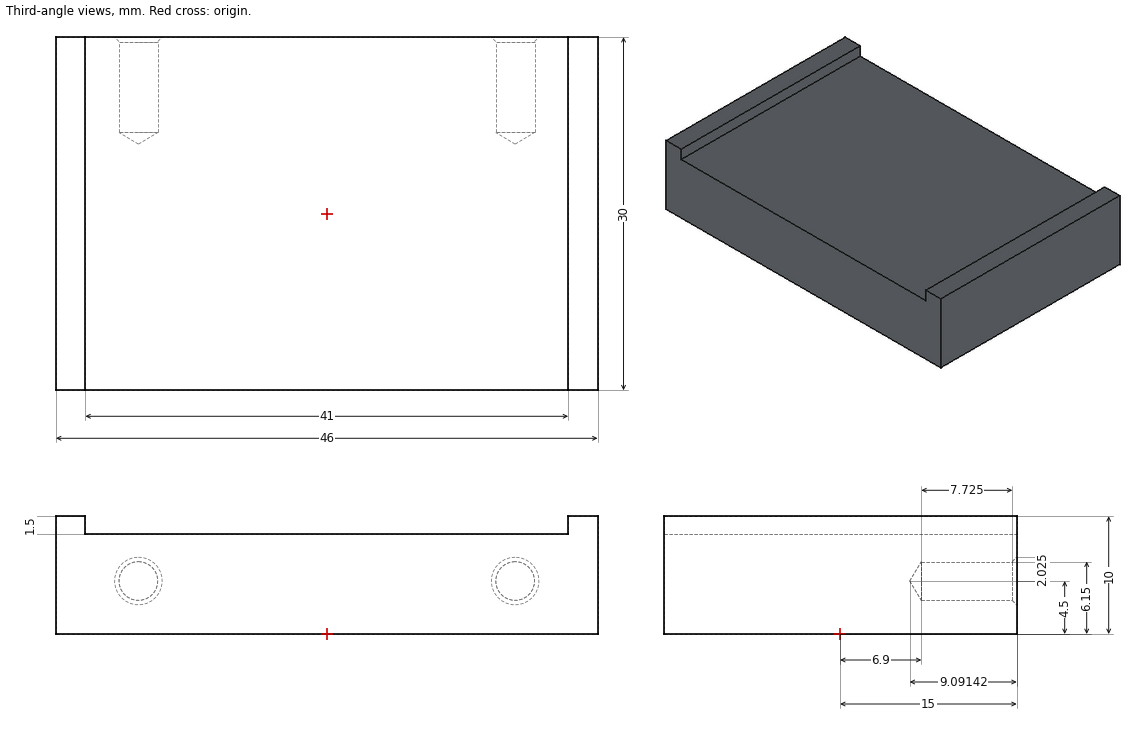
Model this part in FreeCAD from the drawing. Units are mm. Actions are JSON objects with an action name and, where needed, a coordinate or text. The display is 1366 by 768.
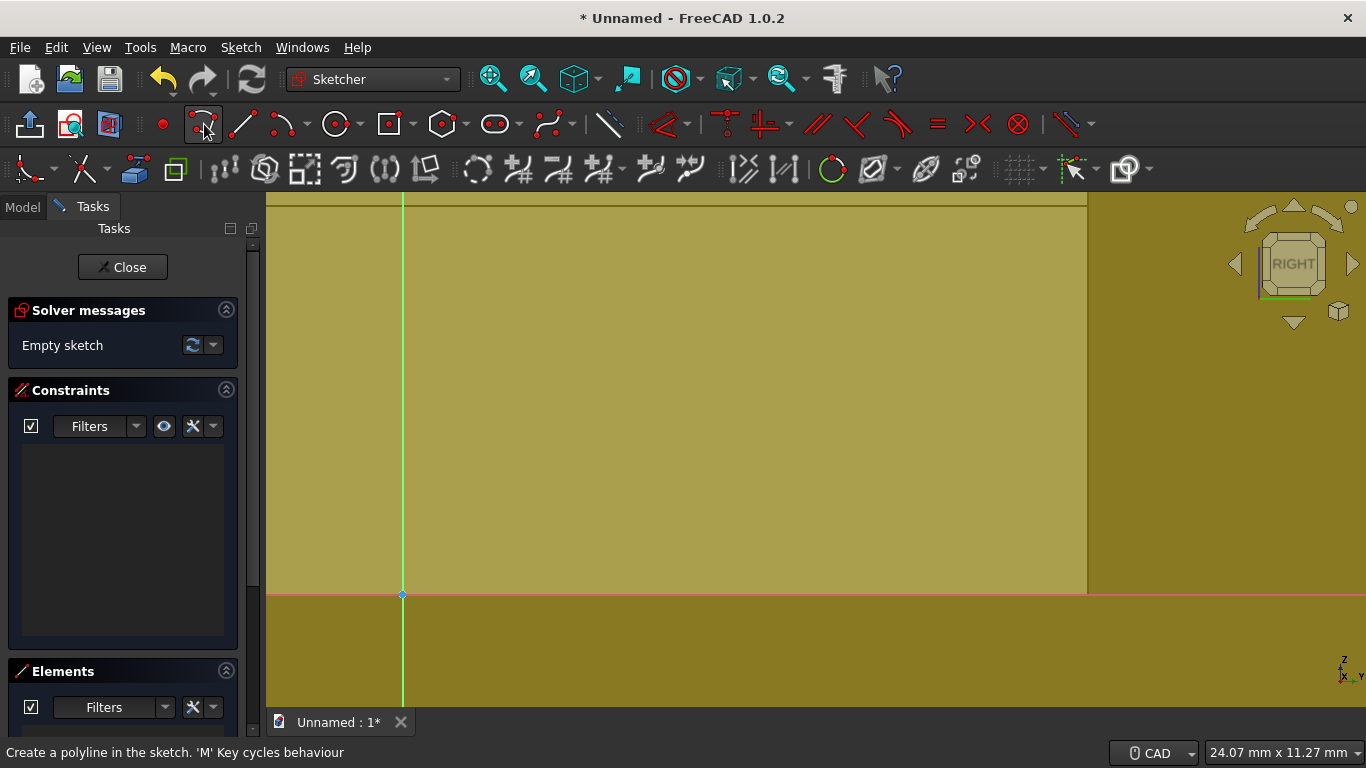
{"action": "left_click", "coordinate": [673, 389]}
{"action": "left_click", "coordinate": [1088, 389]}
{"action": "left_click", "coordinate": [1088, 297]}
{"action": "left_click", "coordinate": [1071, 314]}
{"action": "left_click", "coordinate": [718, 314]}
{"action": "left_click", "coordinate": [673, 390]}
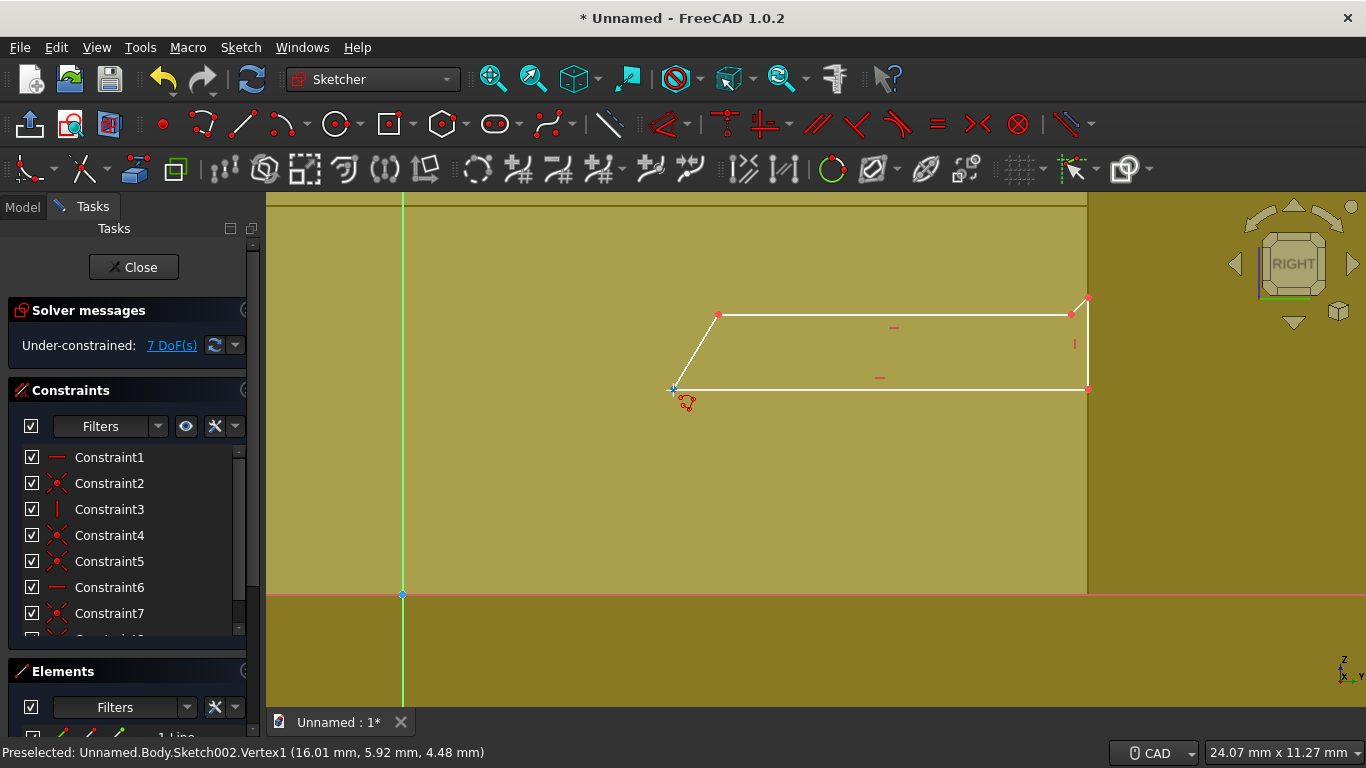
{"action": "left_click", "coordinate": [244, 124]}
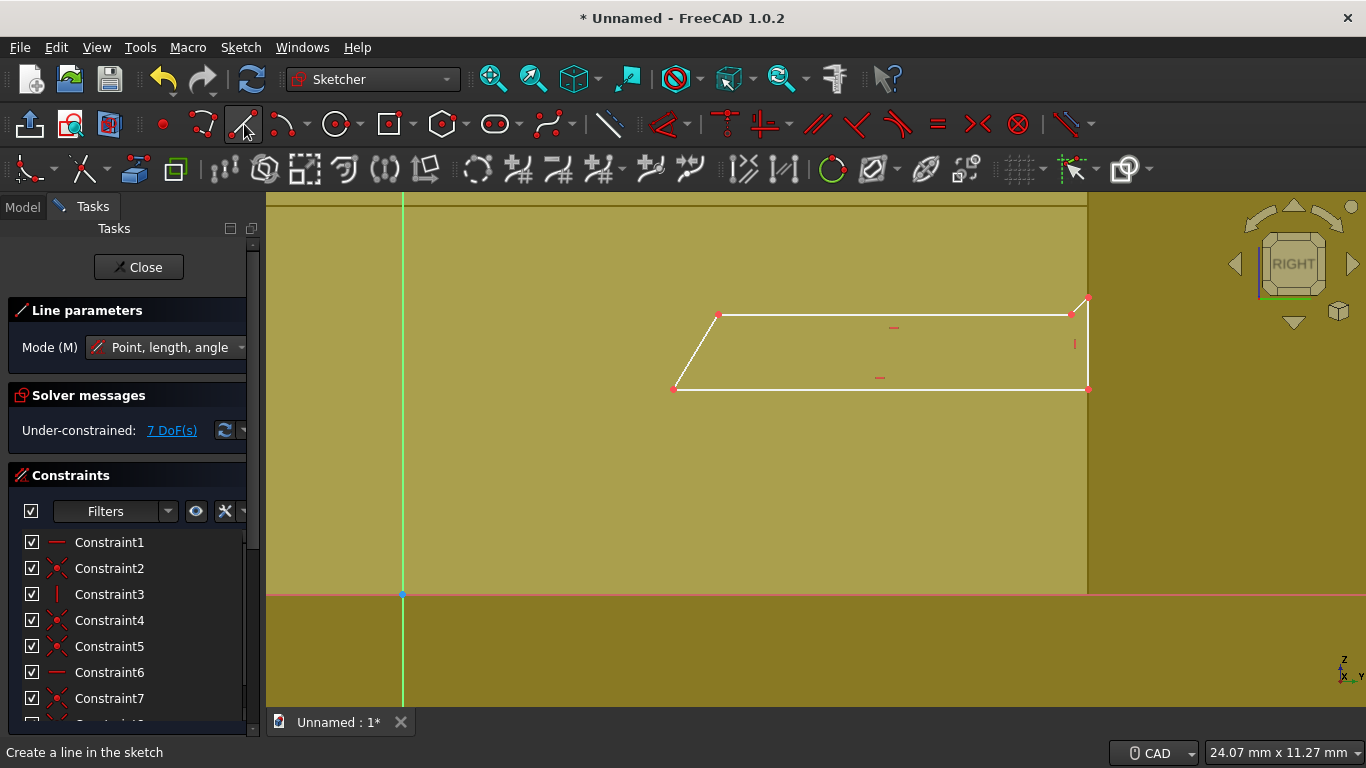
{"action": "left_click", "coordinate": [631, 389]}
{"action": "left_click", "coordinate": [506, 389]}
{"action": "key", "text": "Escape"}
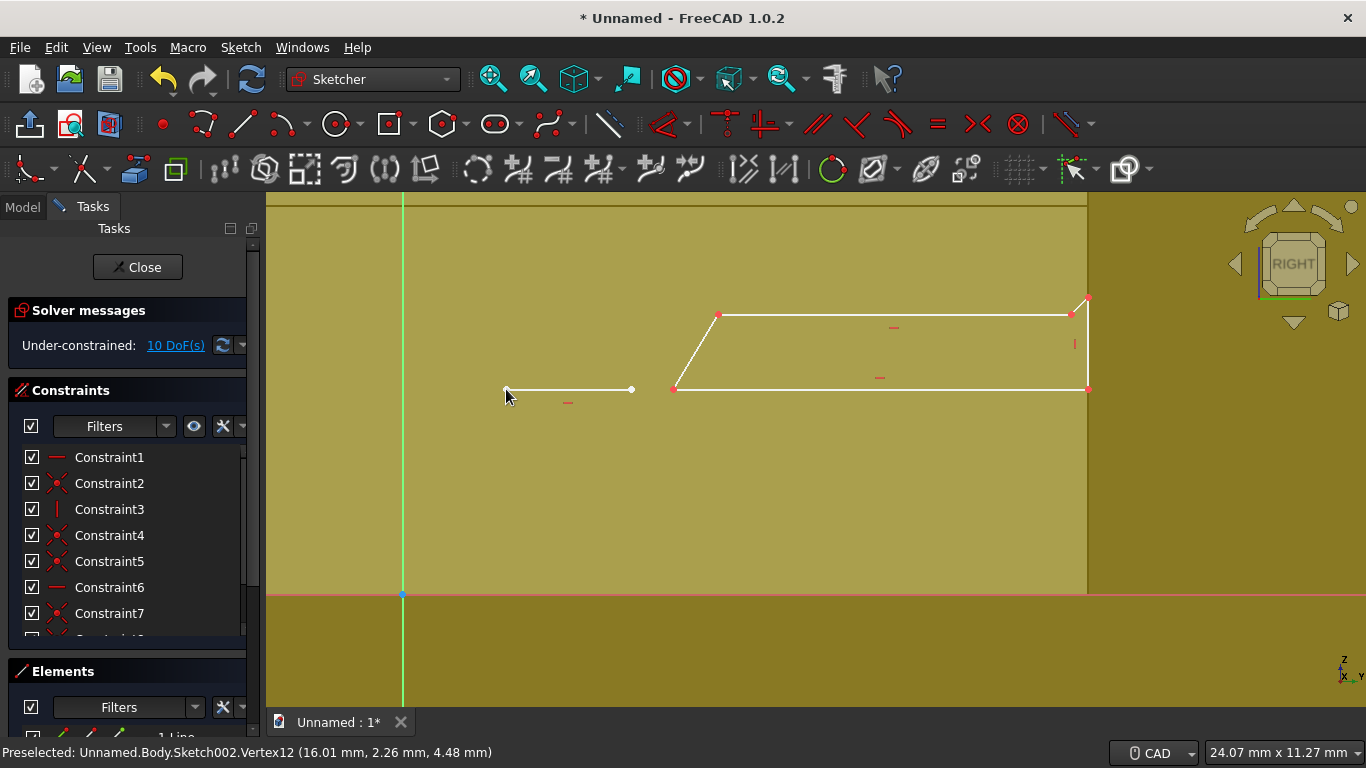
{"action": "left_click", "coordinate": [593, 390]}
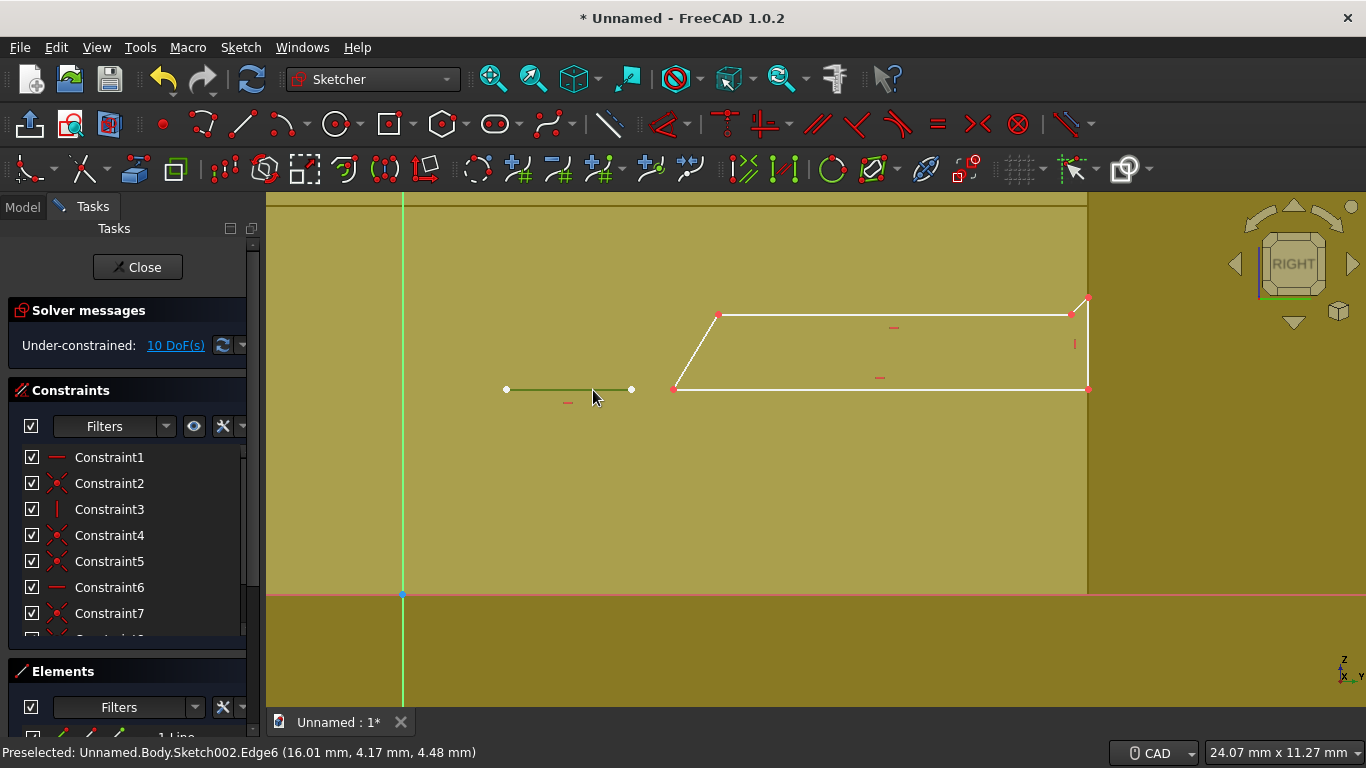
{"action": "left_click", "coordinate": [610, 124]}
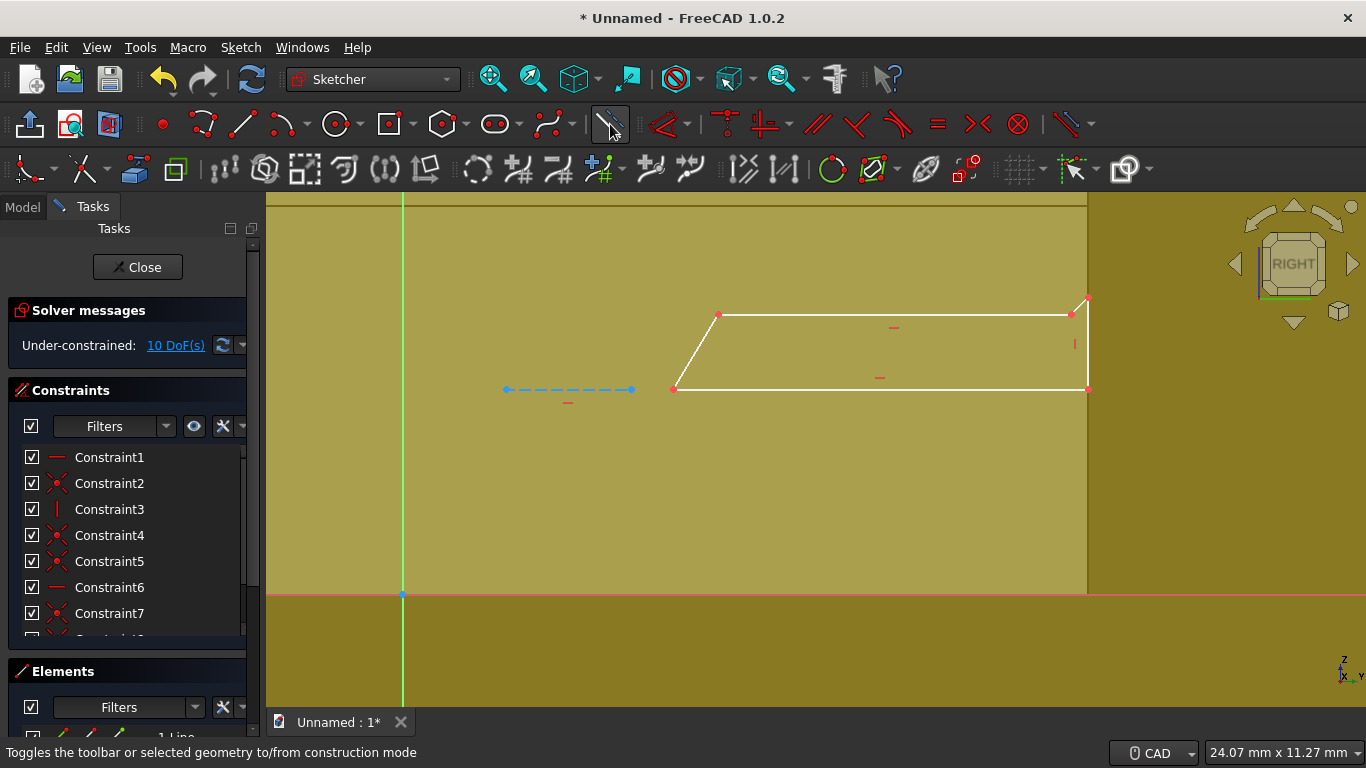
{"action": "left_click", "coordinate": [664, 124]}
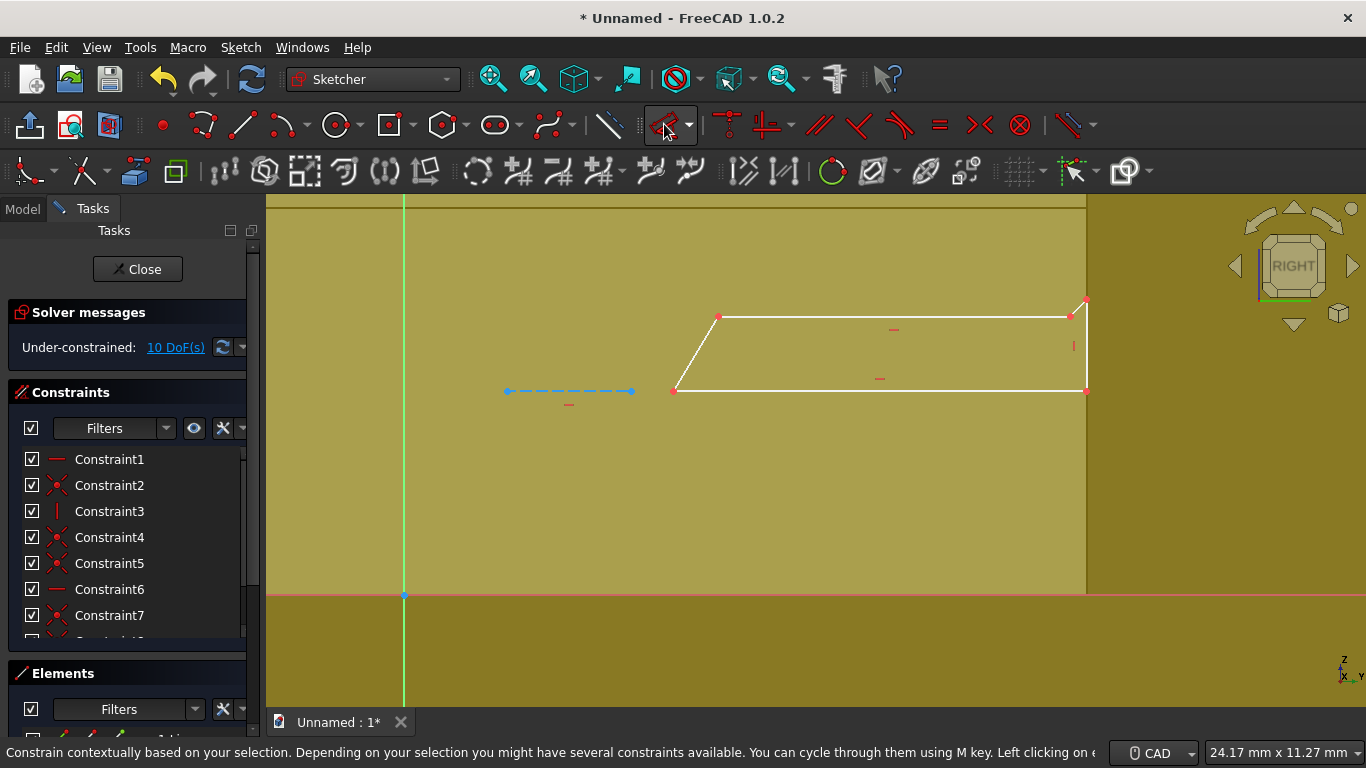
{"action": "left_click", "coordinate": [1087, 391]}
{"action": "left_click", "coordinate": [746, 629]}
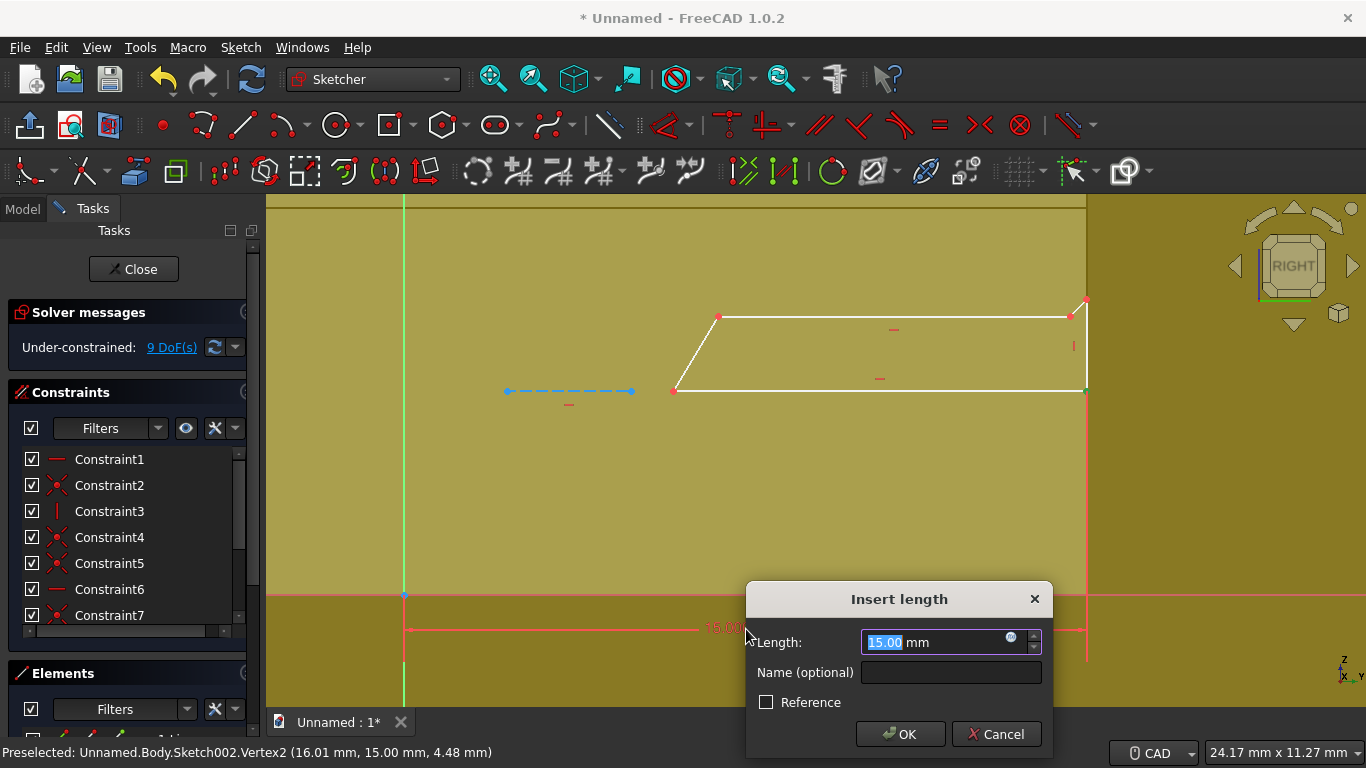
{"action": "type", "text": "15"}
{"action": "key", "text": "Return"}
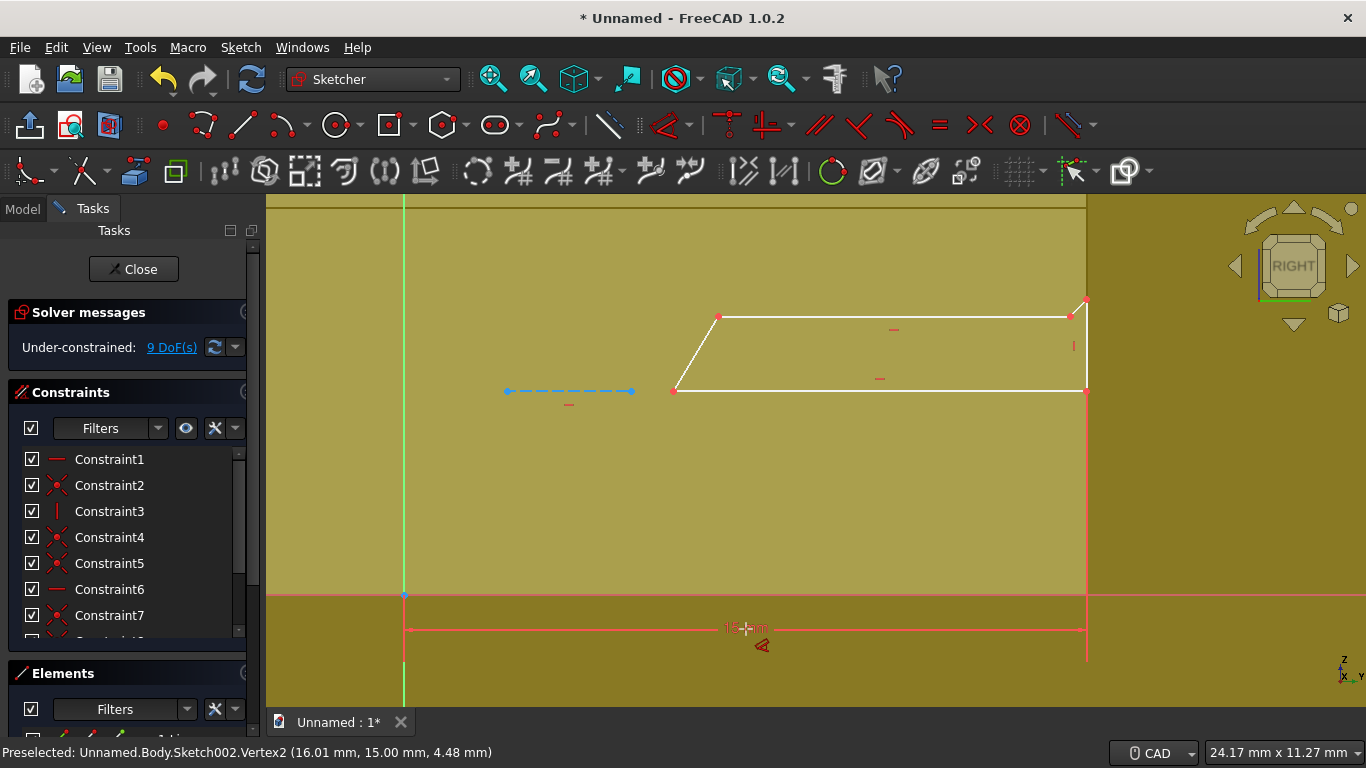
{"action": "left_click", "coordinate": [674, 391]}
{"action": "left_click", "coordinate": [370, 493]}